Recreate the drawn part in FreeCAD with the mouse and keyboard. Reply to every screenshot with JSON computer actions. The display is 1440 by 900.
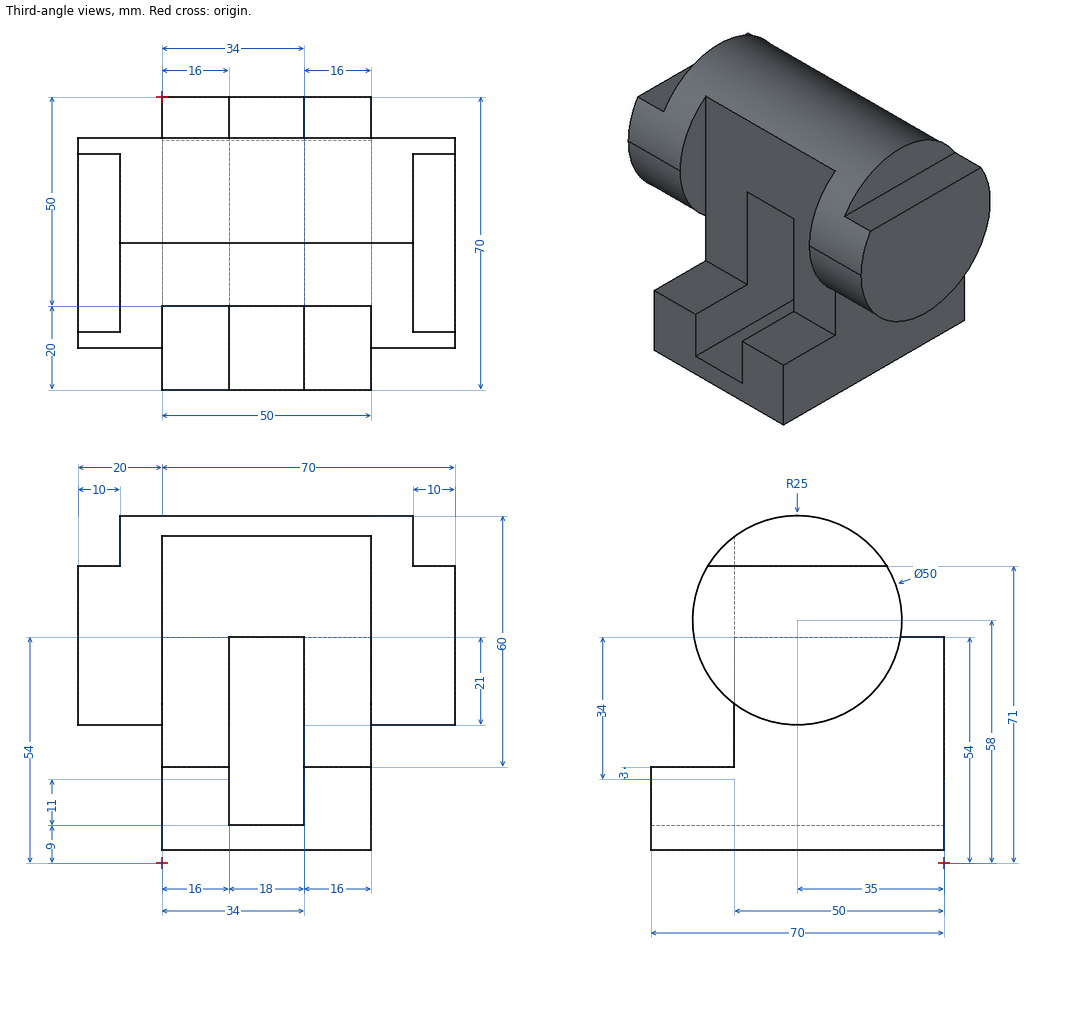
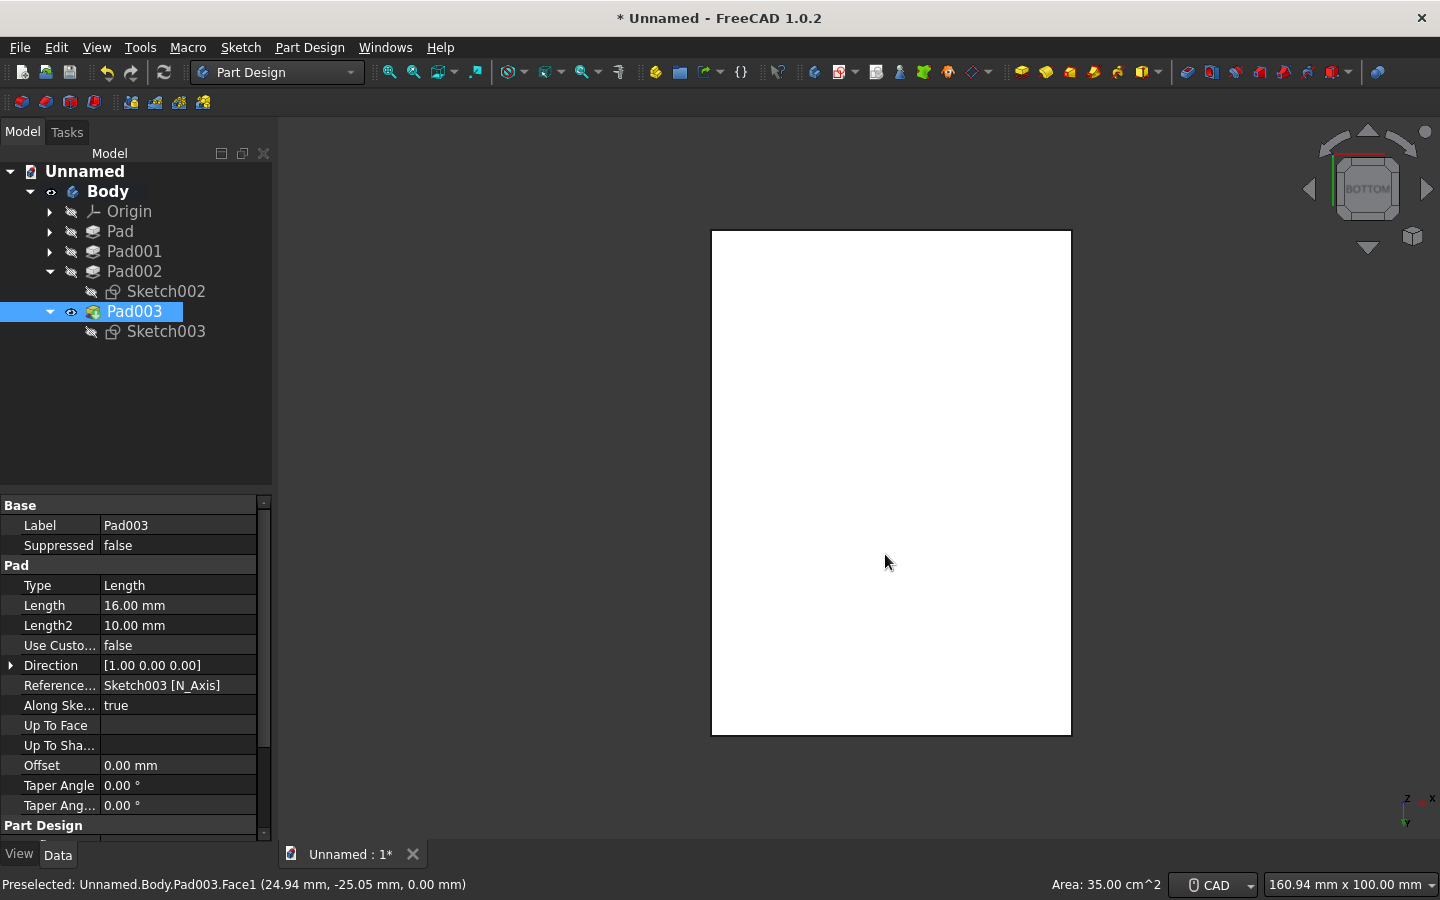
{"action": "left_click", "coordinate": [840, 72]}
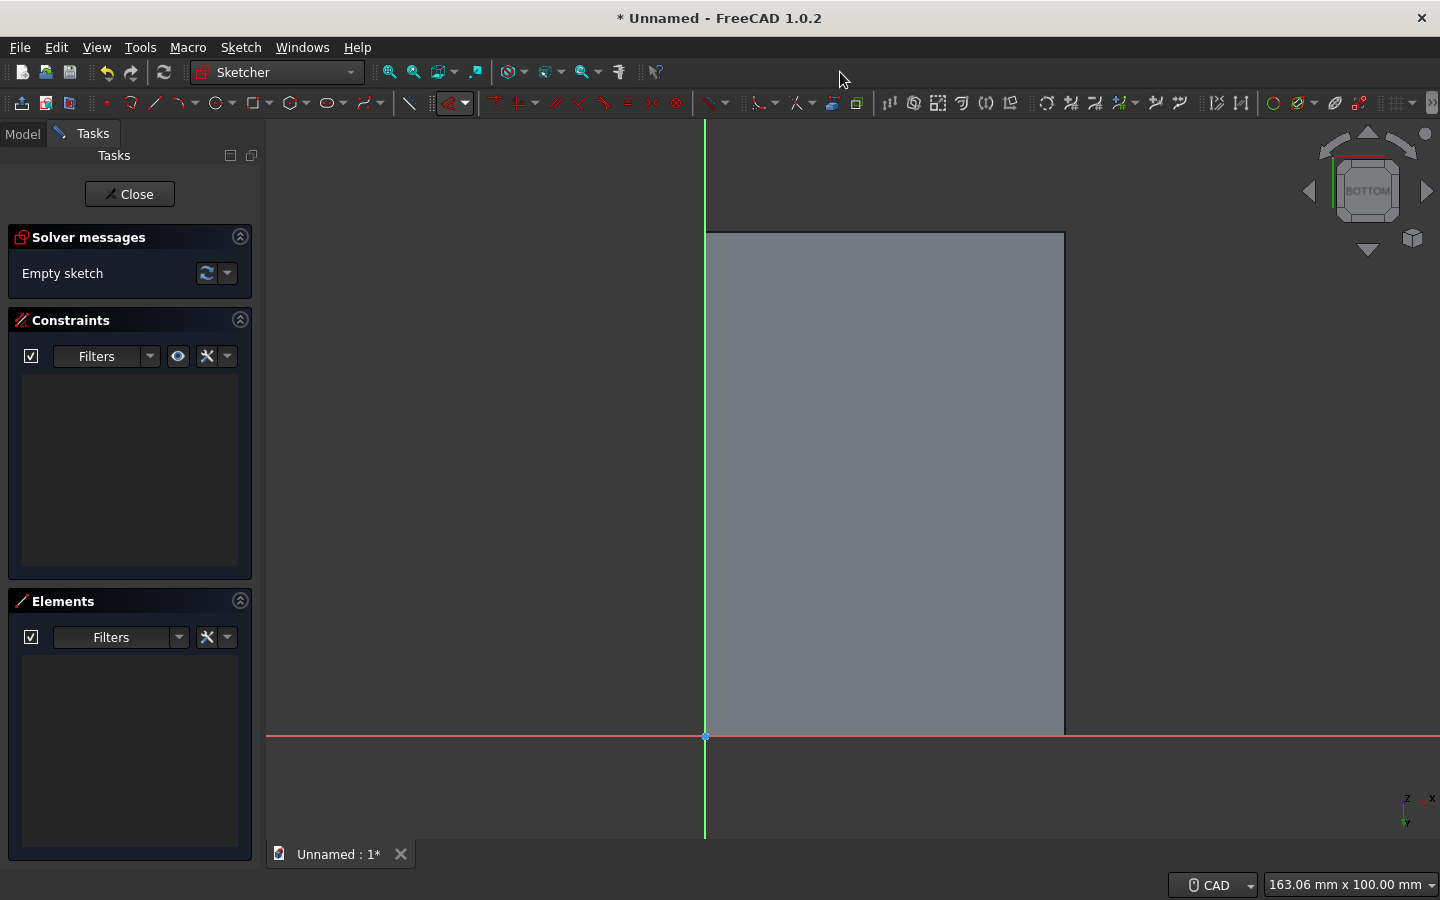
{"action": "key", "text": "g r"}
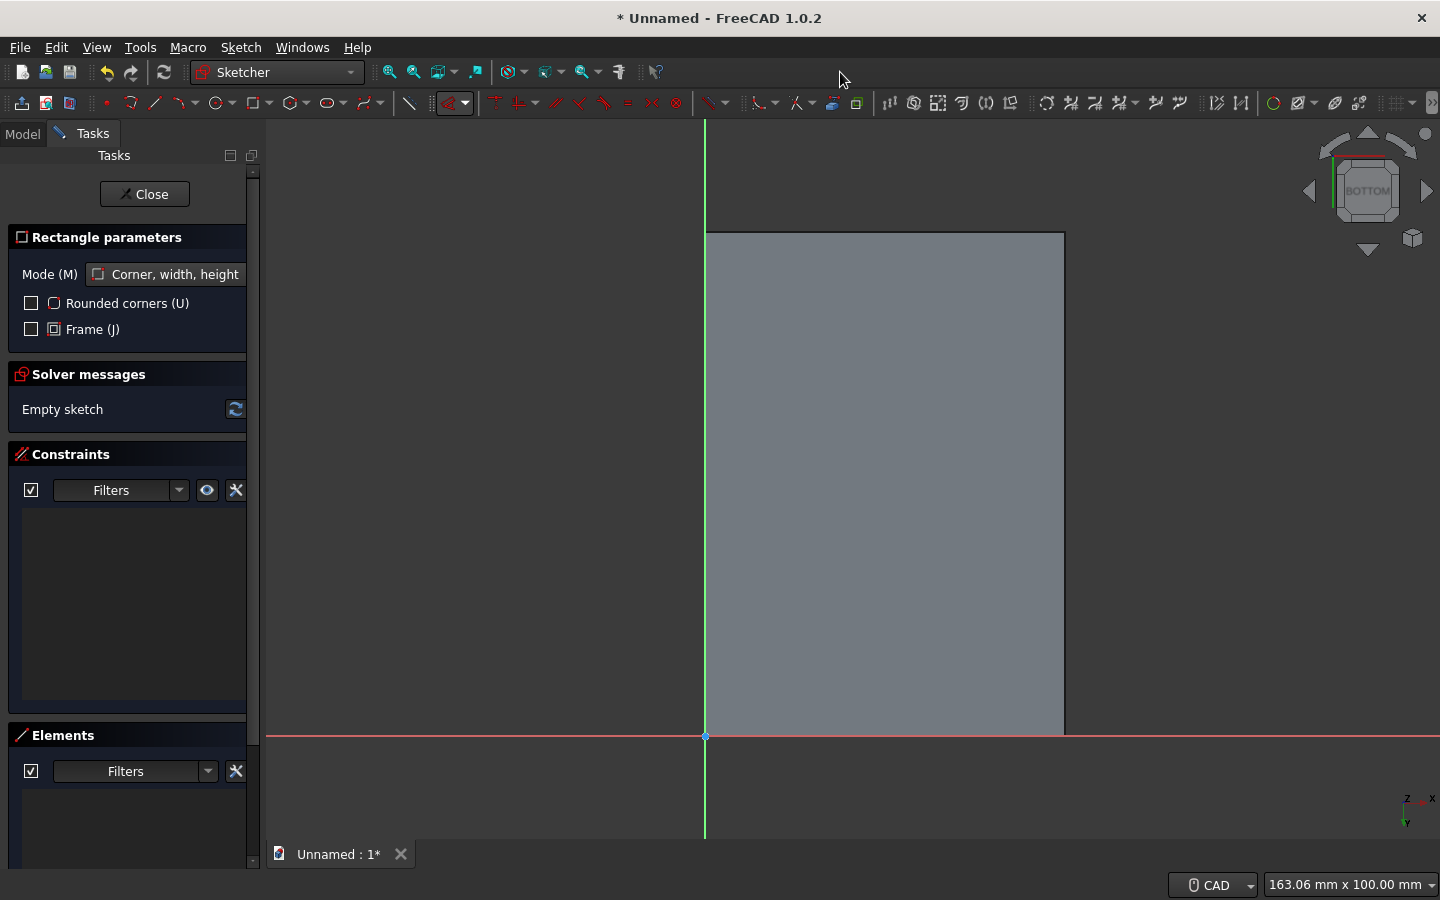
{"action": "left_click", "coordinate": [705, 736]}
{"action": "mouse_move", "coordinate": [1065, 232]}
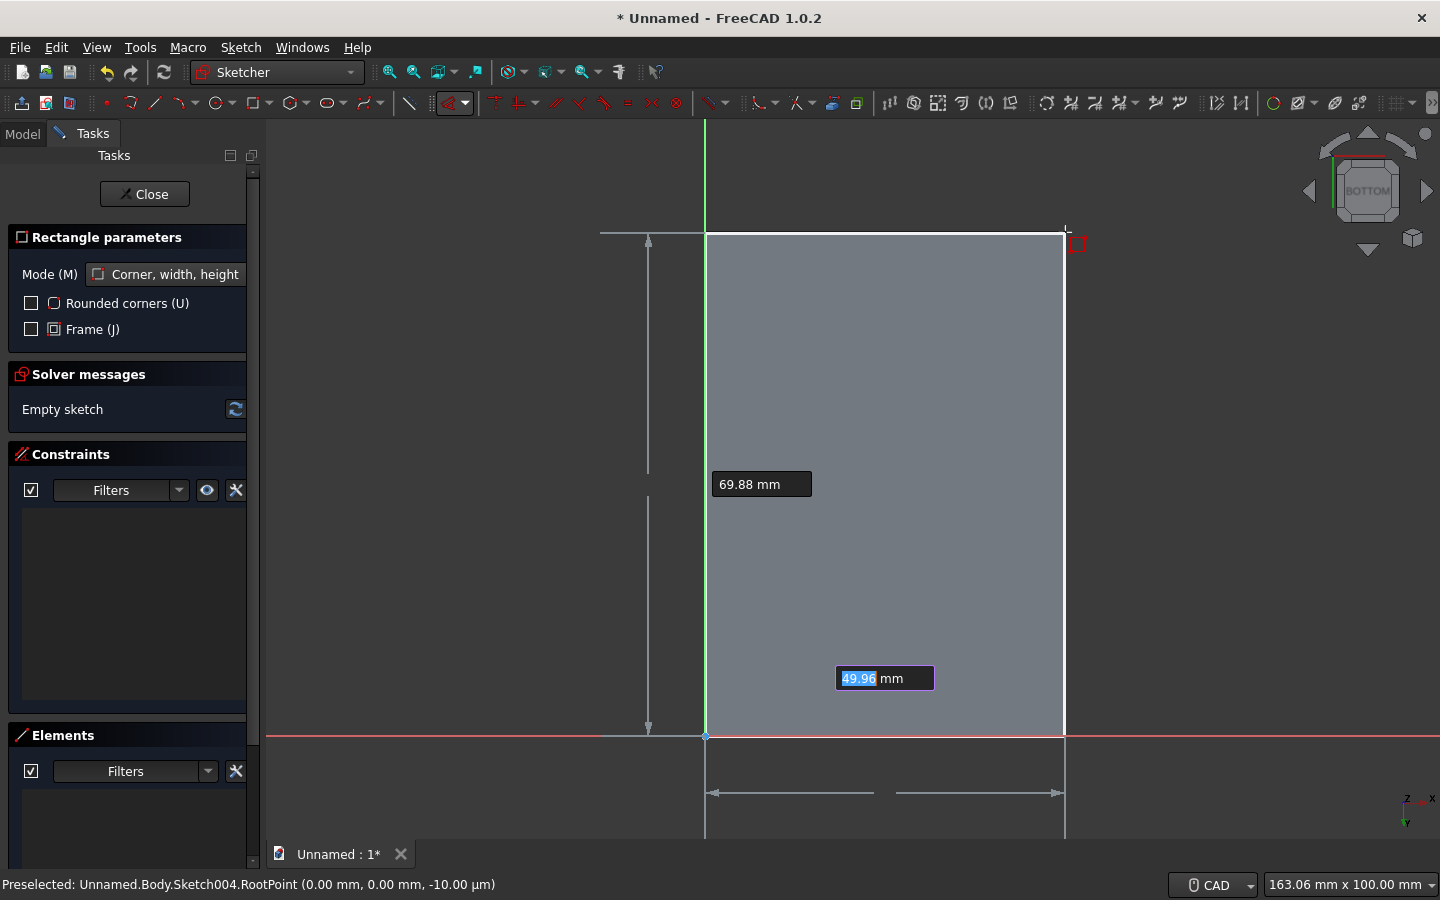
{"action": "type", "text": "50"}
{"action": "key", "text": "Tab"}
{"action": "type", "text": "70"}
{"action": "key", "text": "Return"}
{"action": "key", "text": "Escape"}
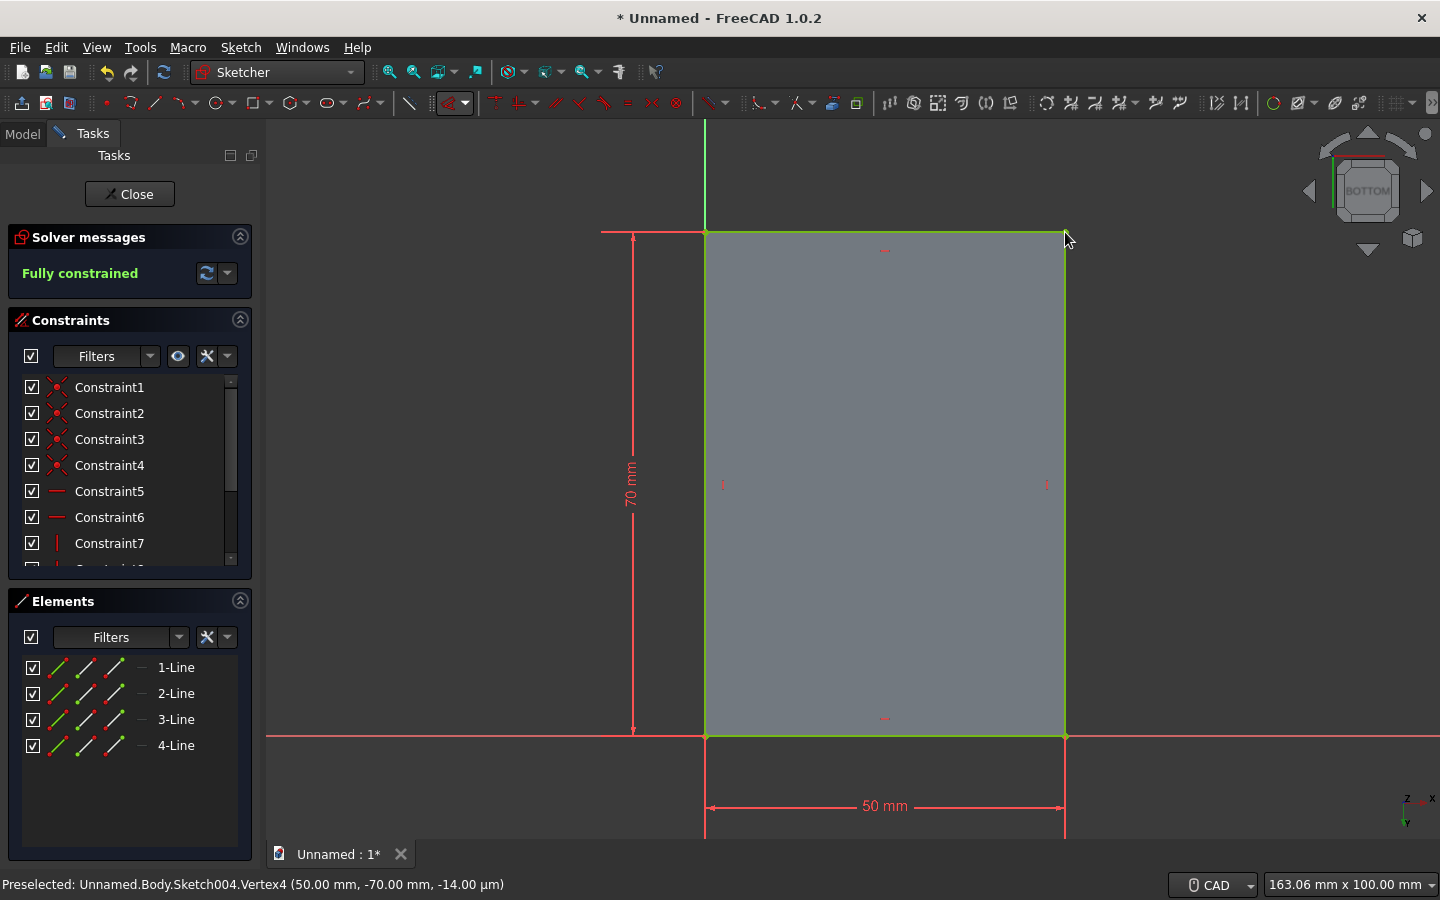
{"action": "left_click", "coordinate": [130, 194]}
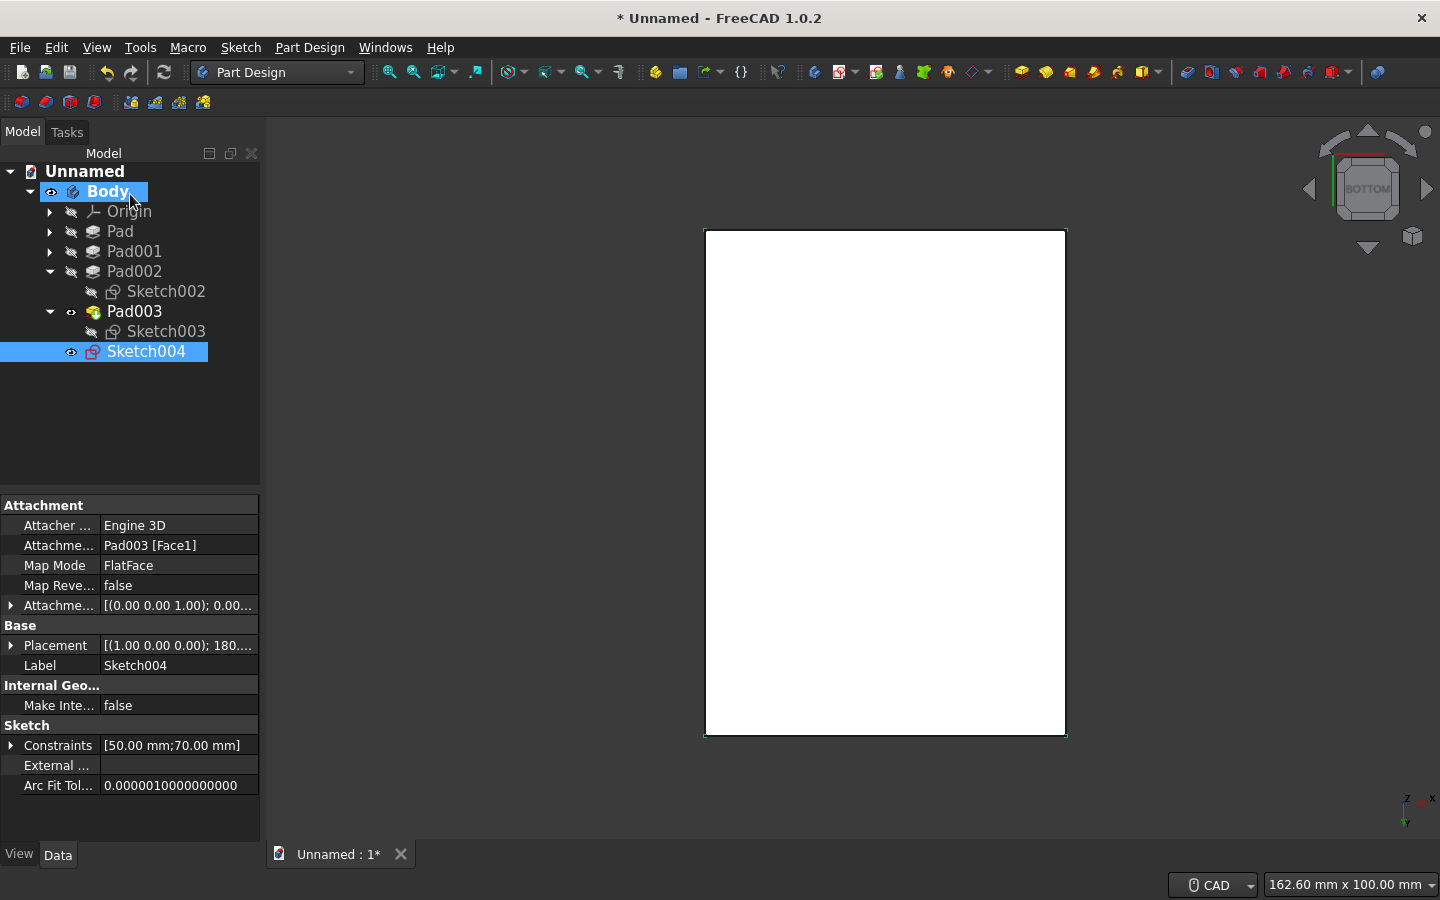
{"action": "left_click", "coordinate": [1188, 72]}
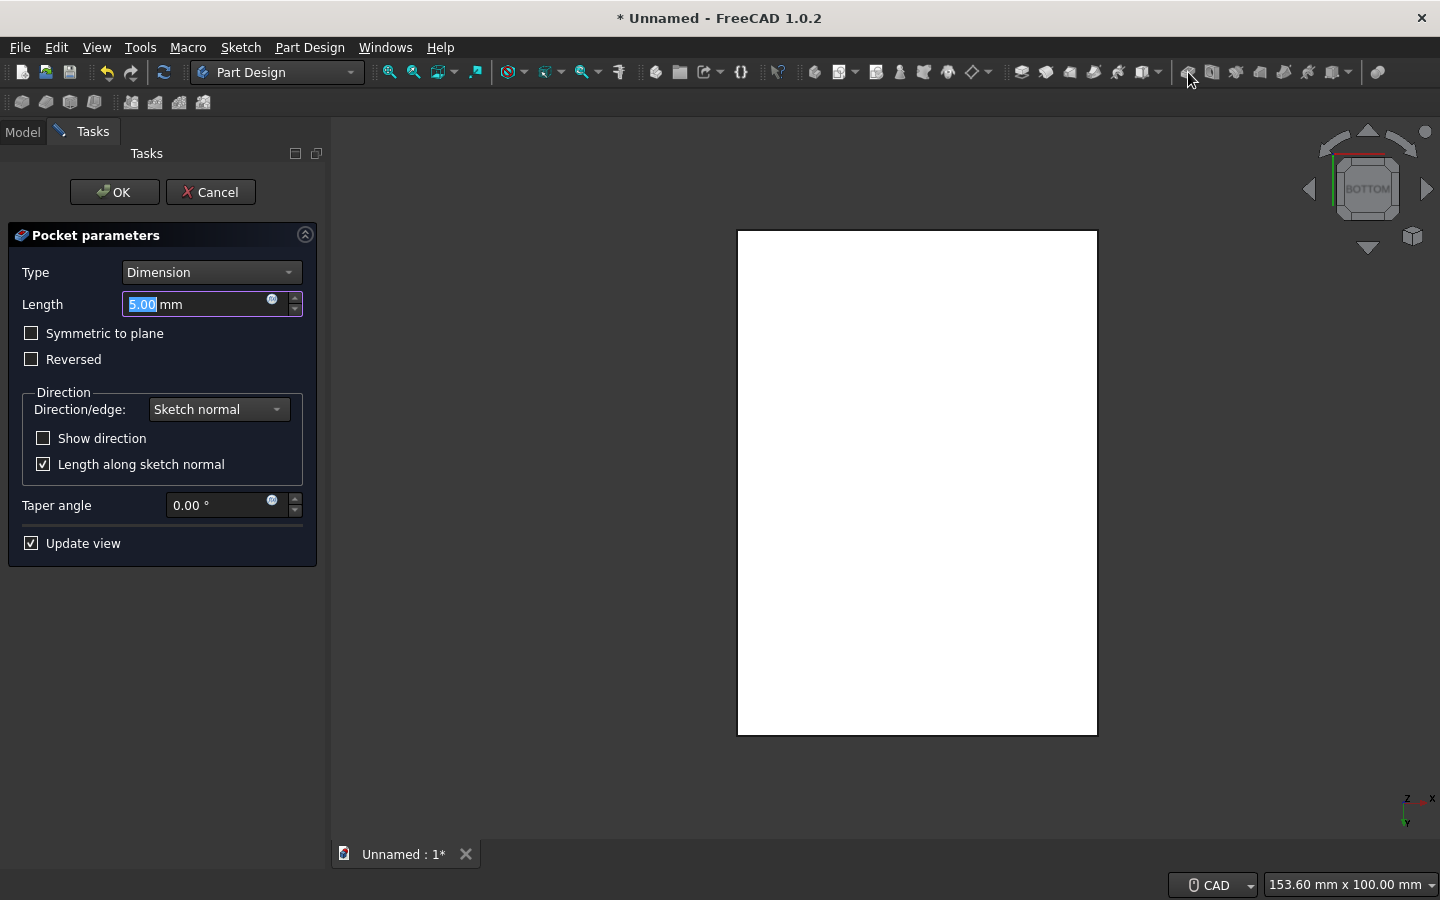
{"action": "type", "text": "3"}
{"action": "key", "text": "Tab"}